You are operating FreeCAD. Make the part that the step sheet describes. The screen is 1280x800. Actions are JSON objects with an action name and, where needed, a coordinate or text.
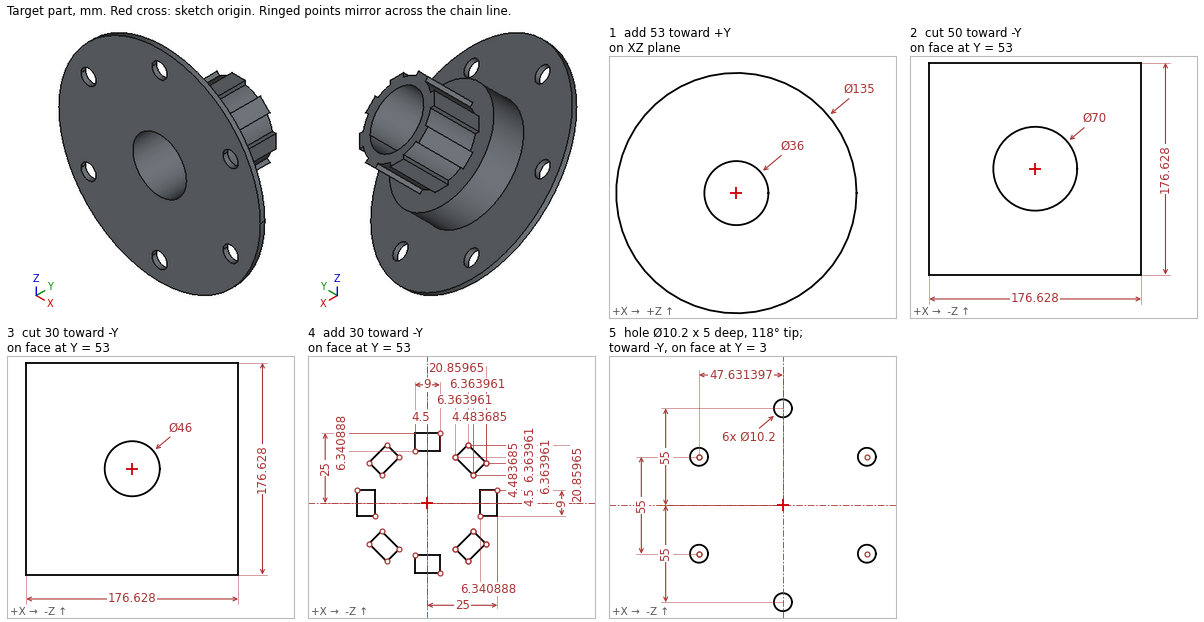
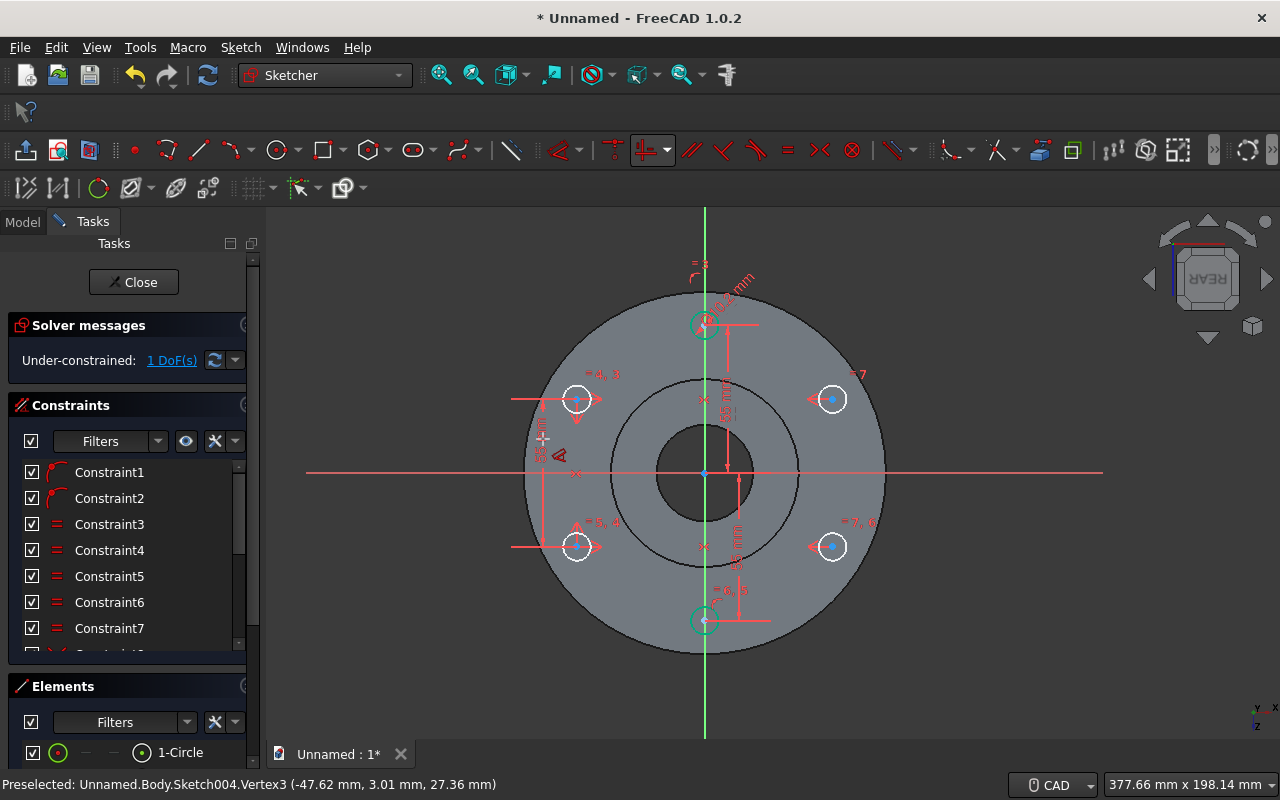
{"action": "left_click", "coordinate": [577, 399]}
{"action": "left_click", "coordinate": [641, 365]}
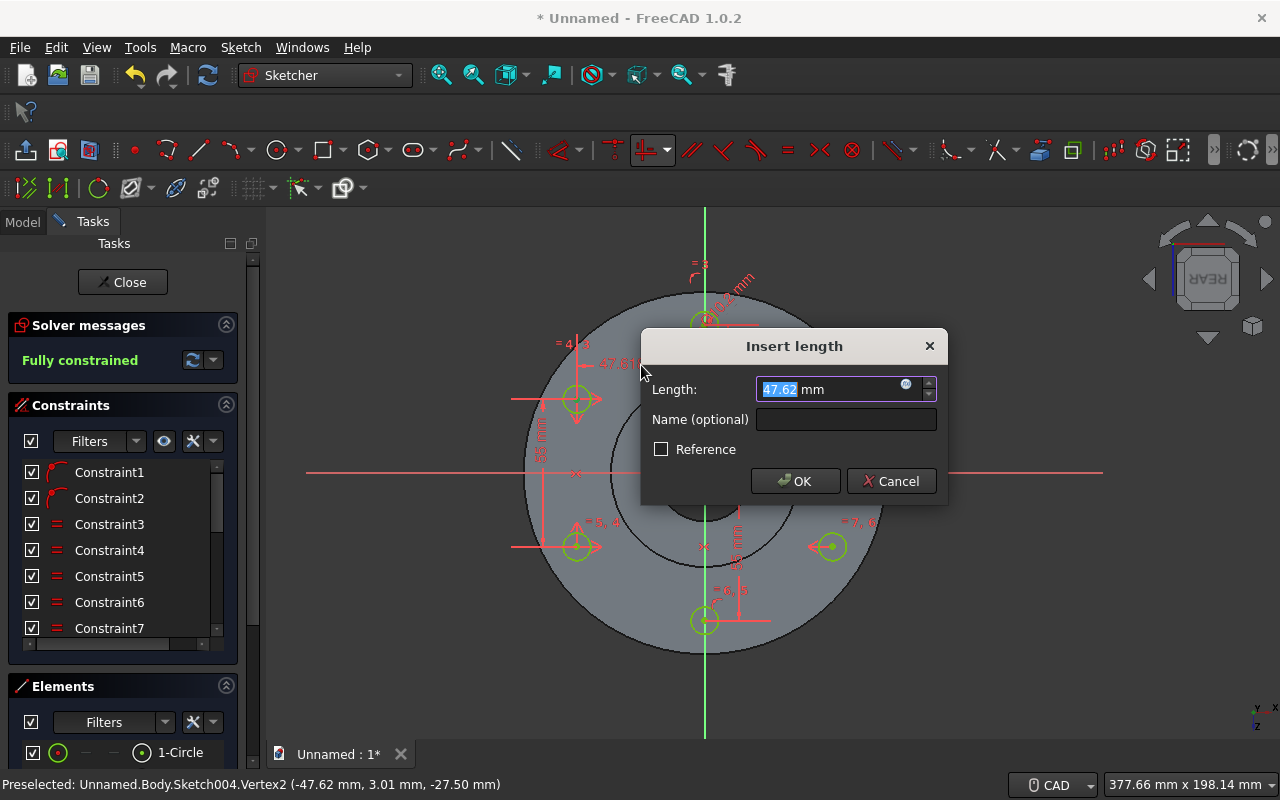
{"action": "type", "text": "47.631397"}
{"action": "key", "text": "Return"}
{"action": "key", "text": "Escape"}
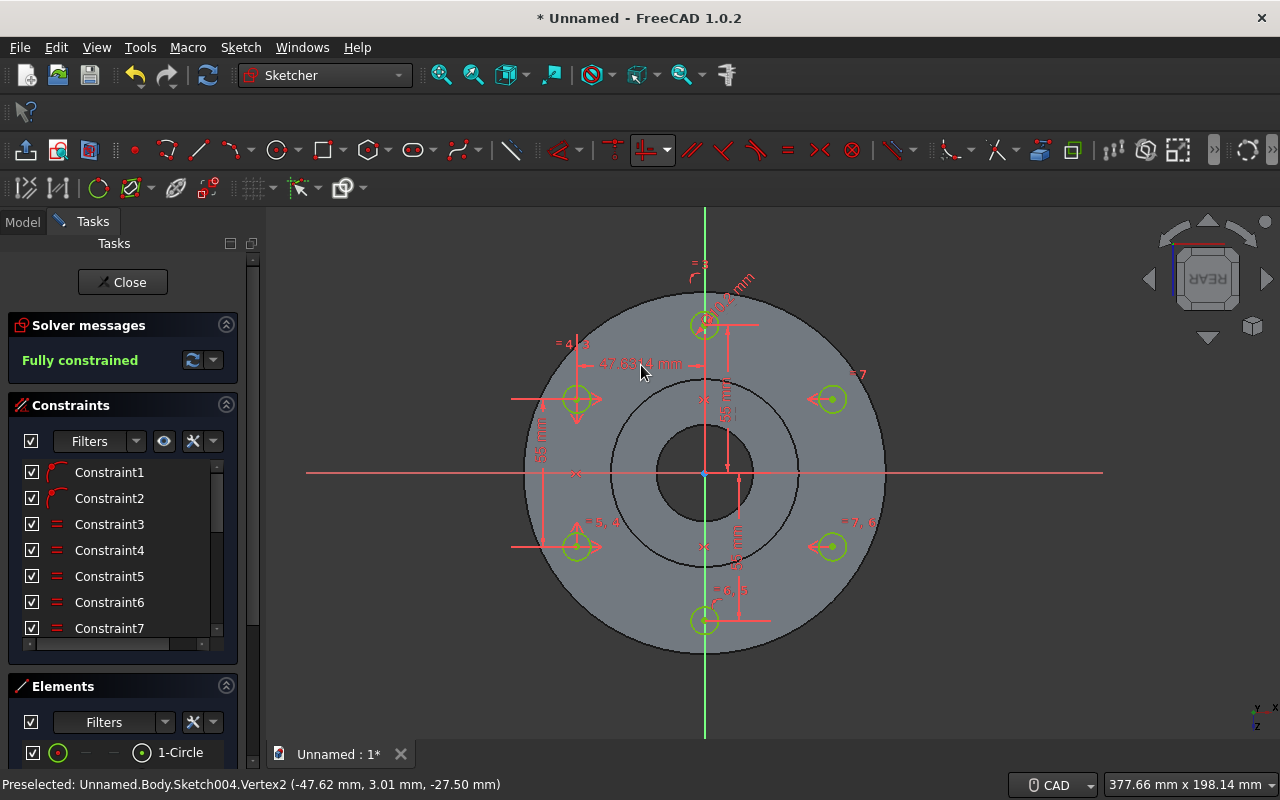
{"action": "left_click", "coordinate": [123, 282]}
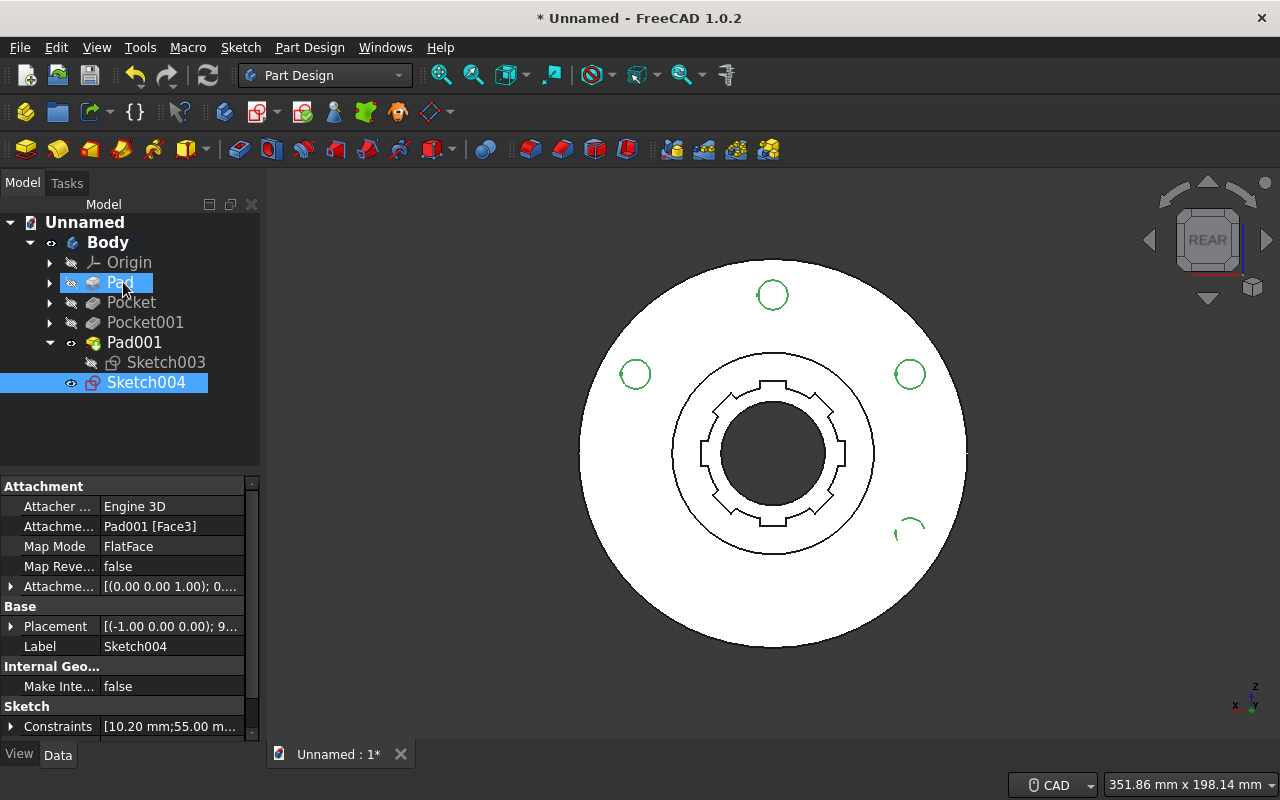
{"action": "left_click", "coordinate": [272, 150]}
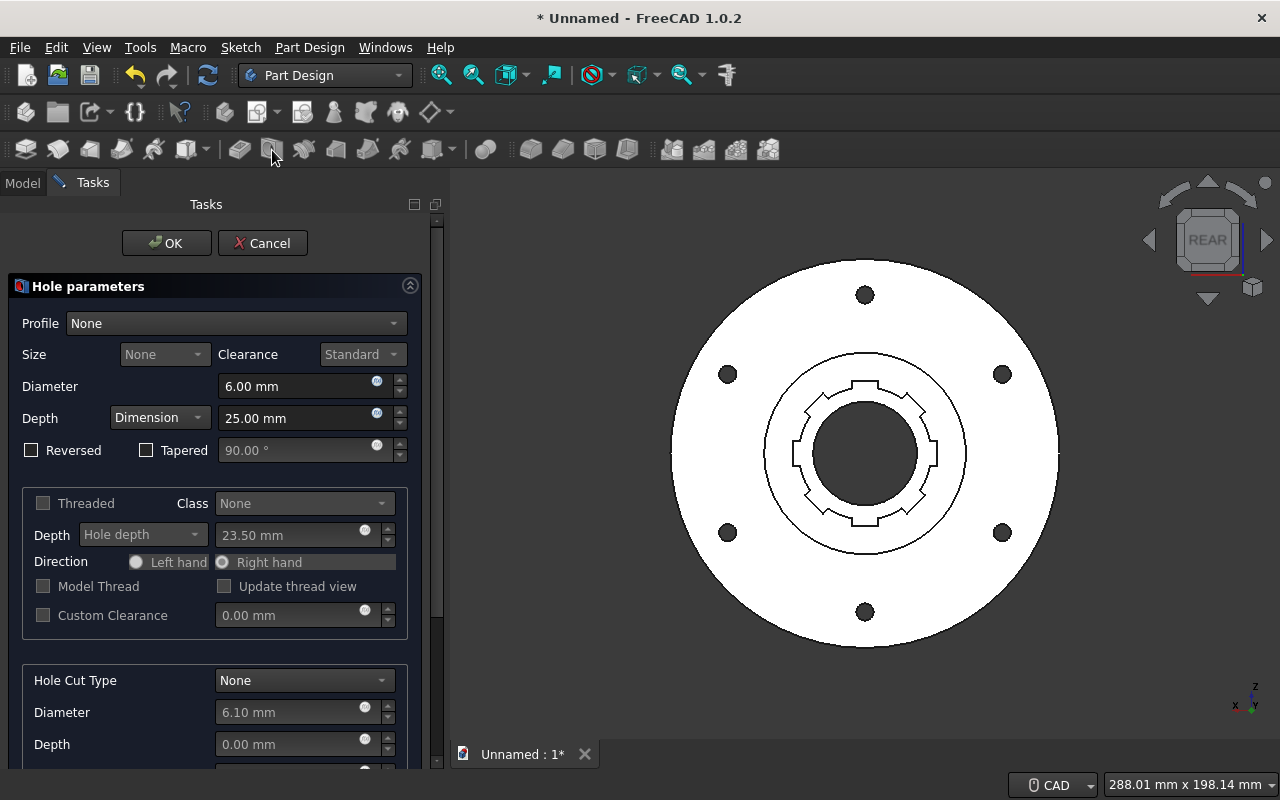
{"action": "triple_click", "coordinate": [305, 386]}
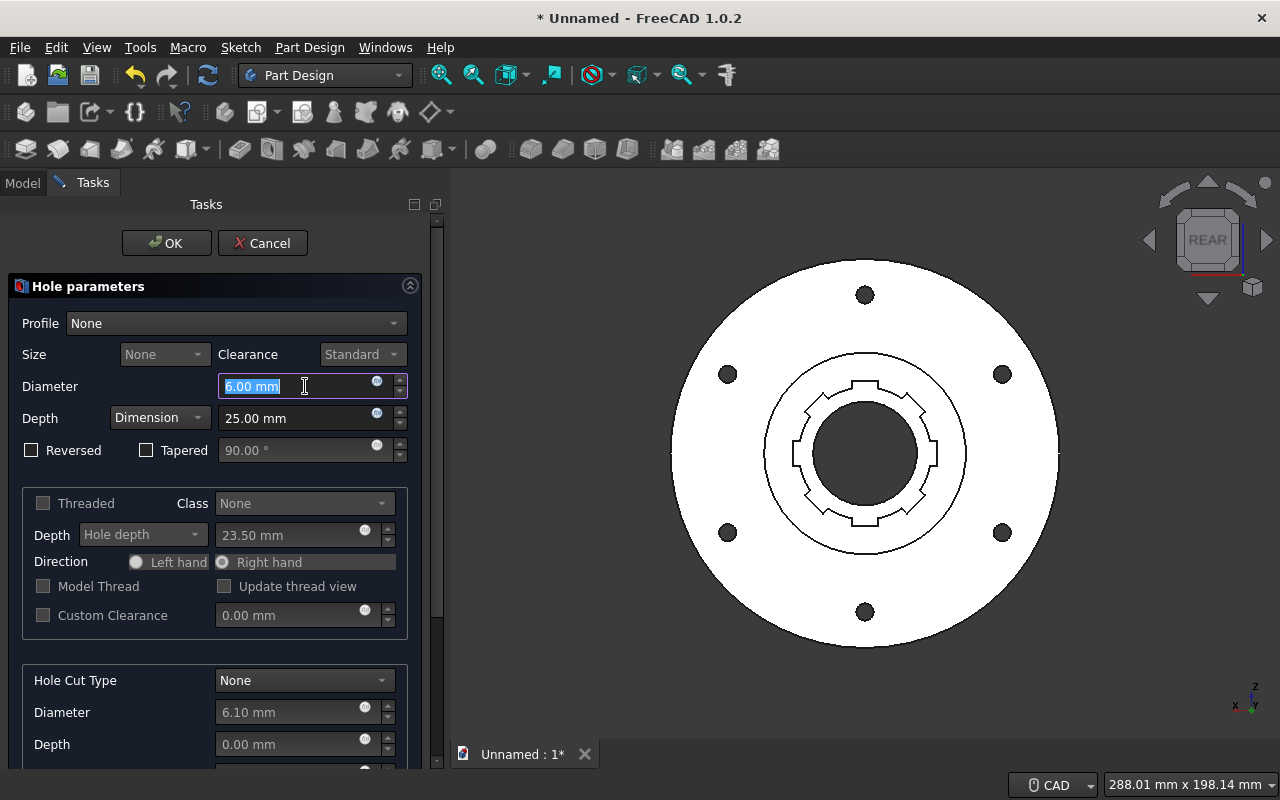
{"action": "type", "text": "10.2"}
{"action": "key", "text": "Tab"}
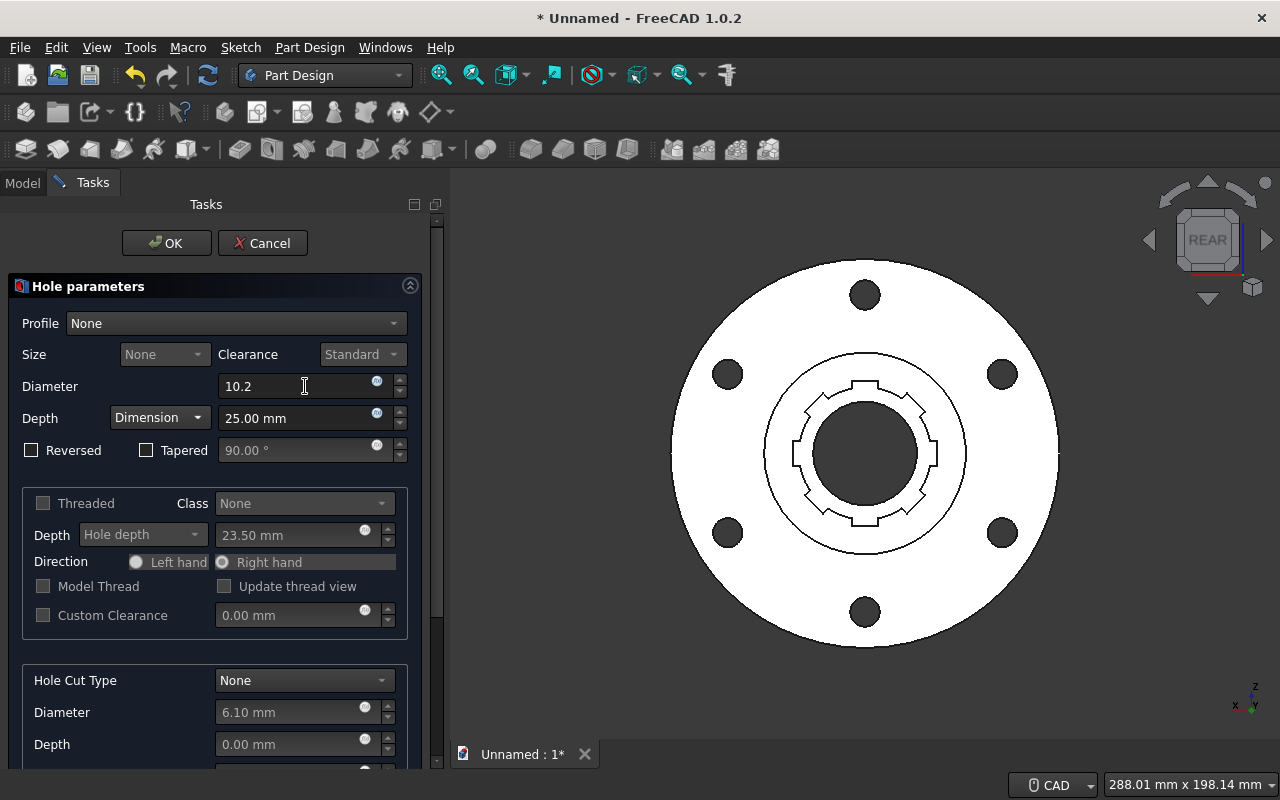
{"action": "triple_click", "coordinate": [305, 418]}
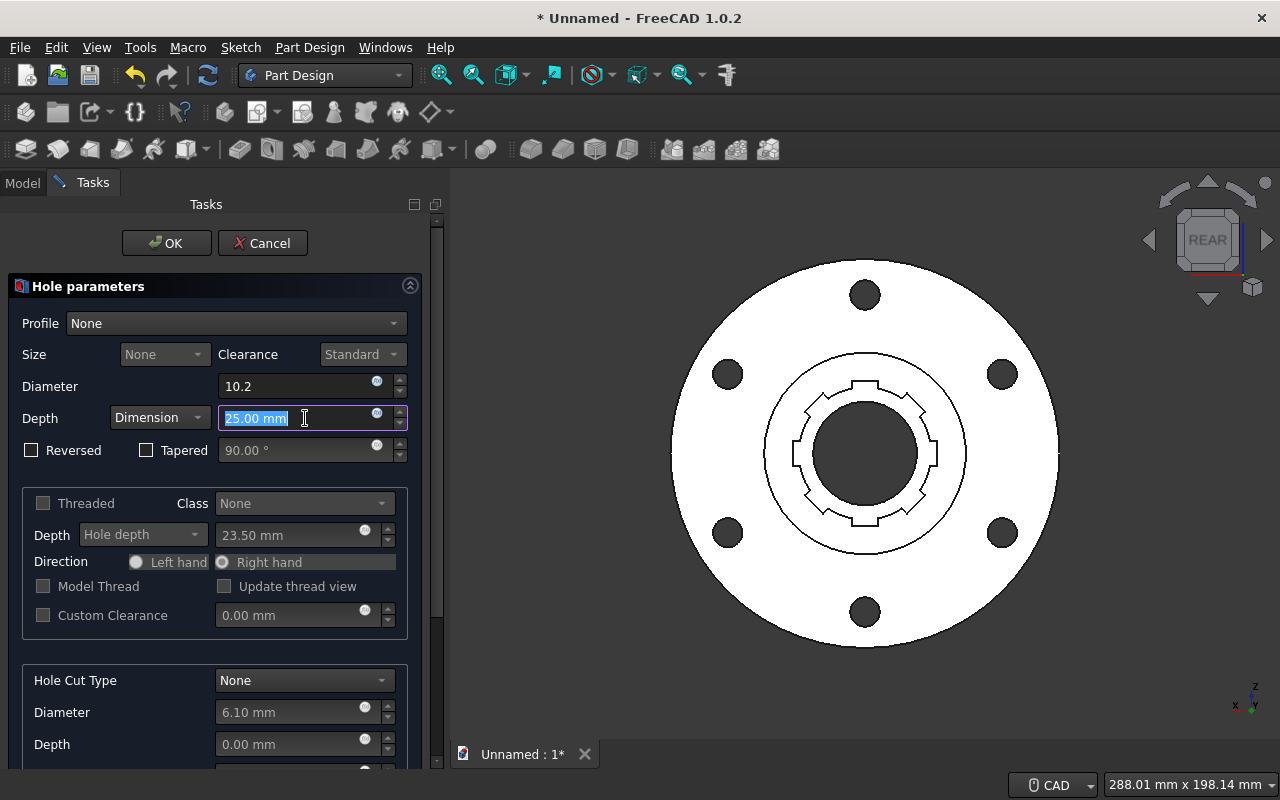
{"action": "type", "text": "5"}
{"action": "key", "text": "Tab"}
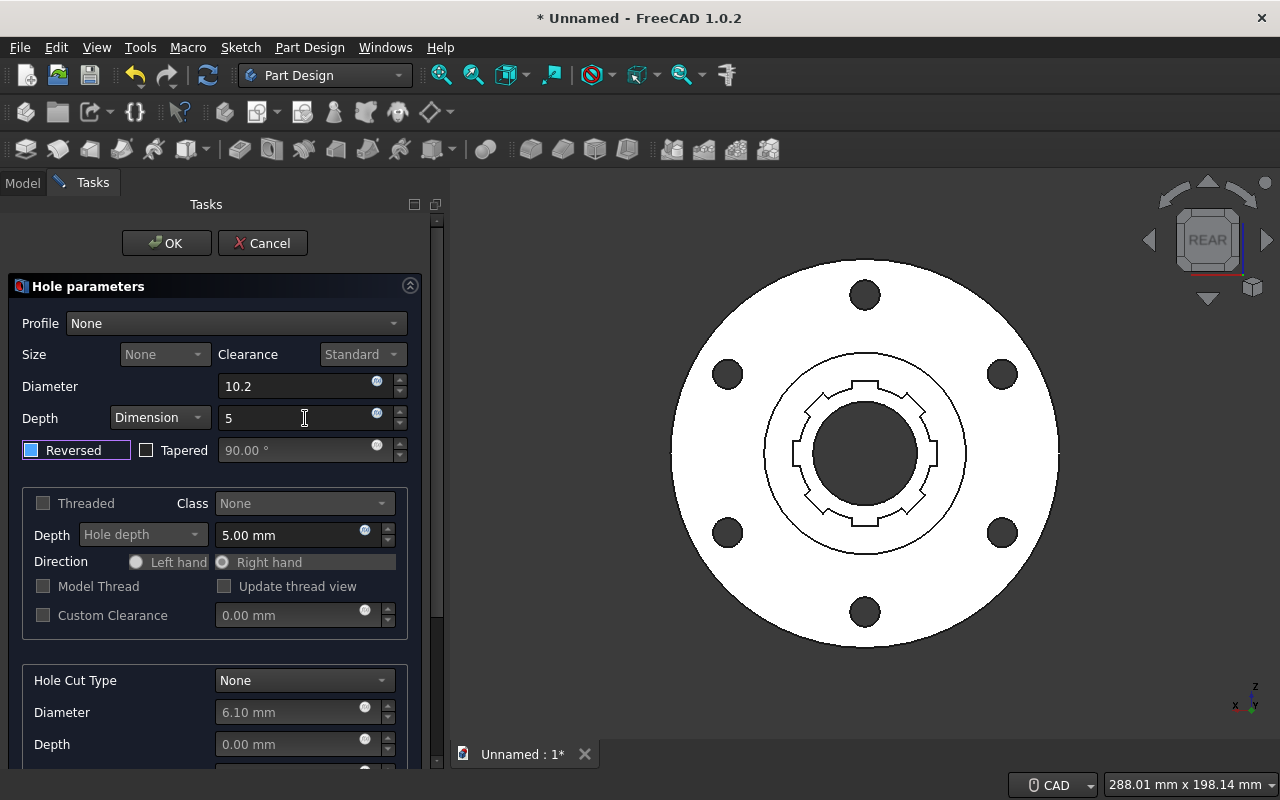
{"action": "left_click", "coordinate": [167, 243]}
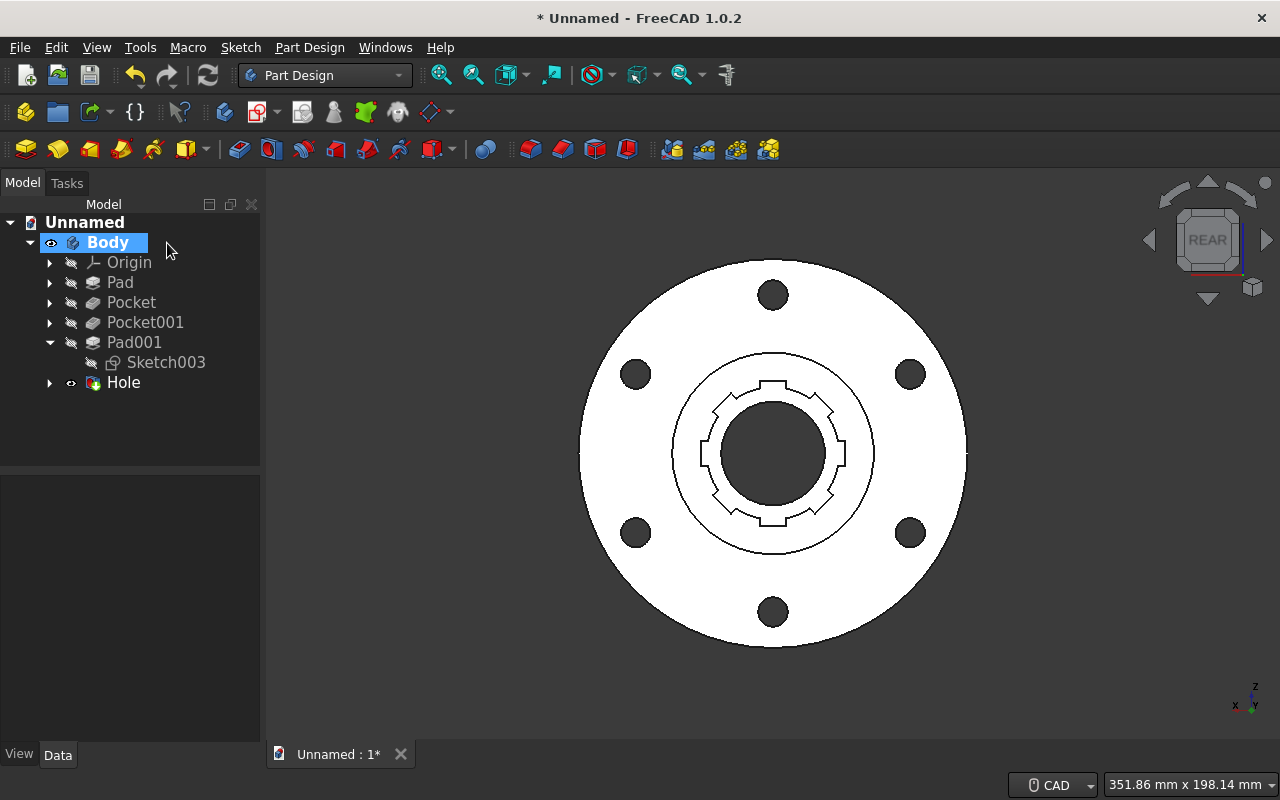
{"action": "key", "text": "0"}